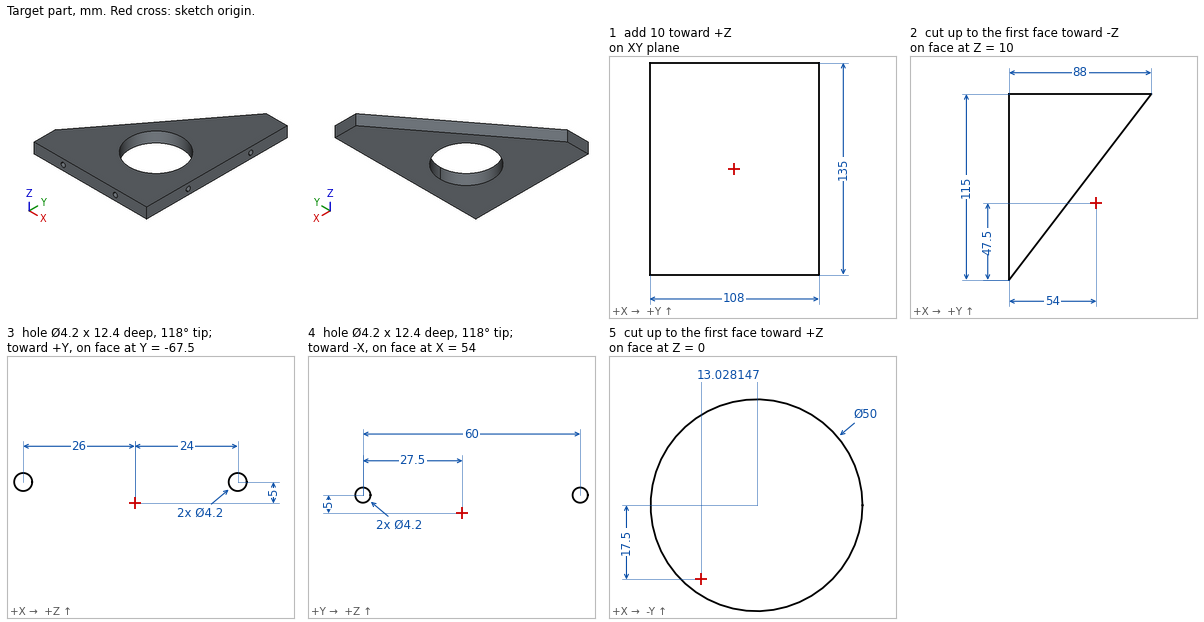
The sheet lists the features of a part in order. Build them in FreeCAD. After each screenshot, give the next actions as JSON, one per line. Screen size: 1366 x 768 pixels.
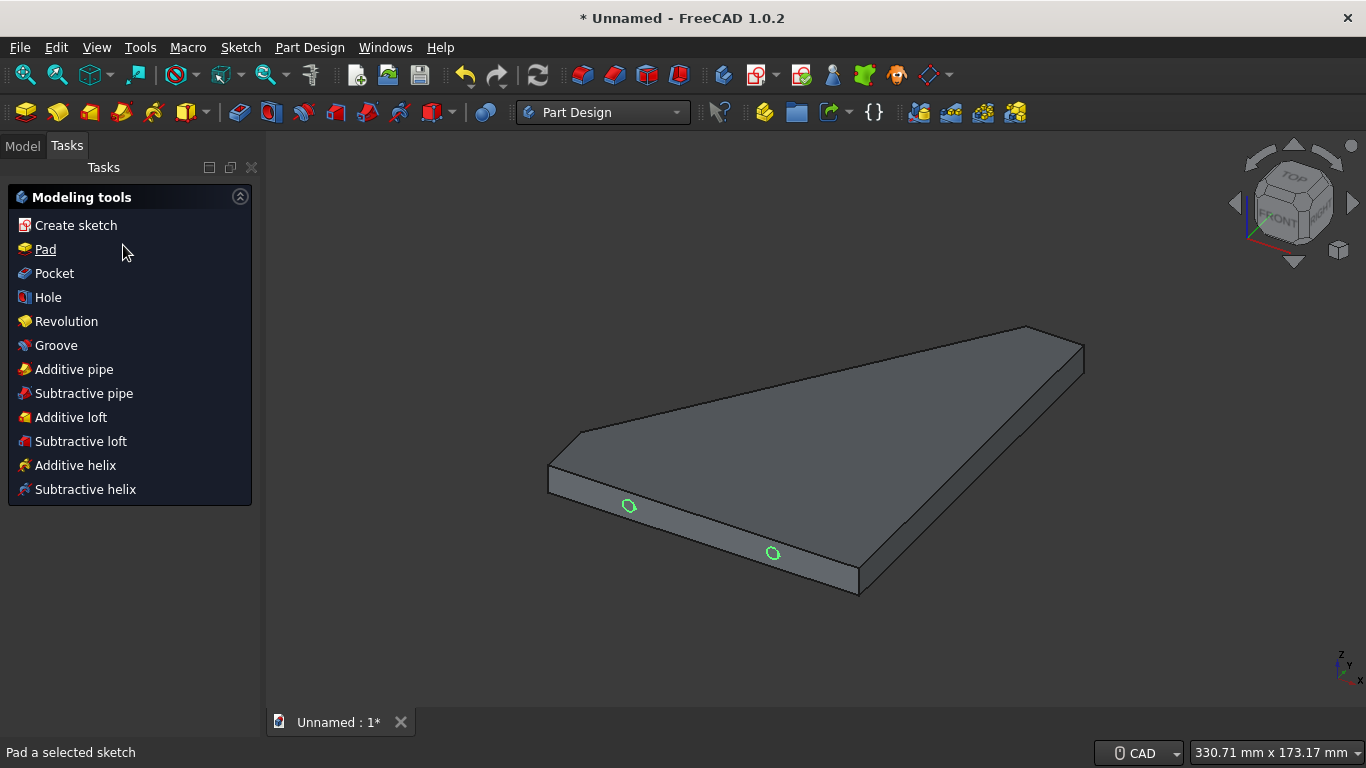
{"action": "left_click", "coordinate": [272, 112]}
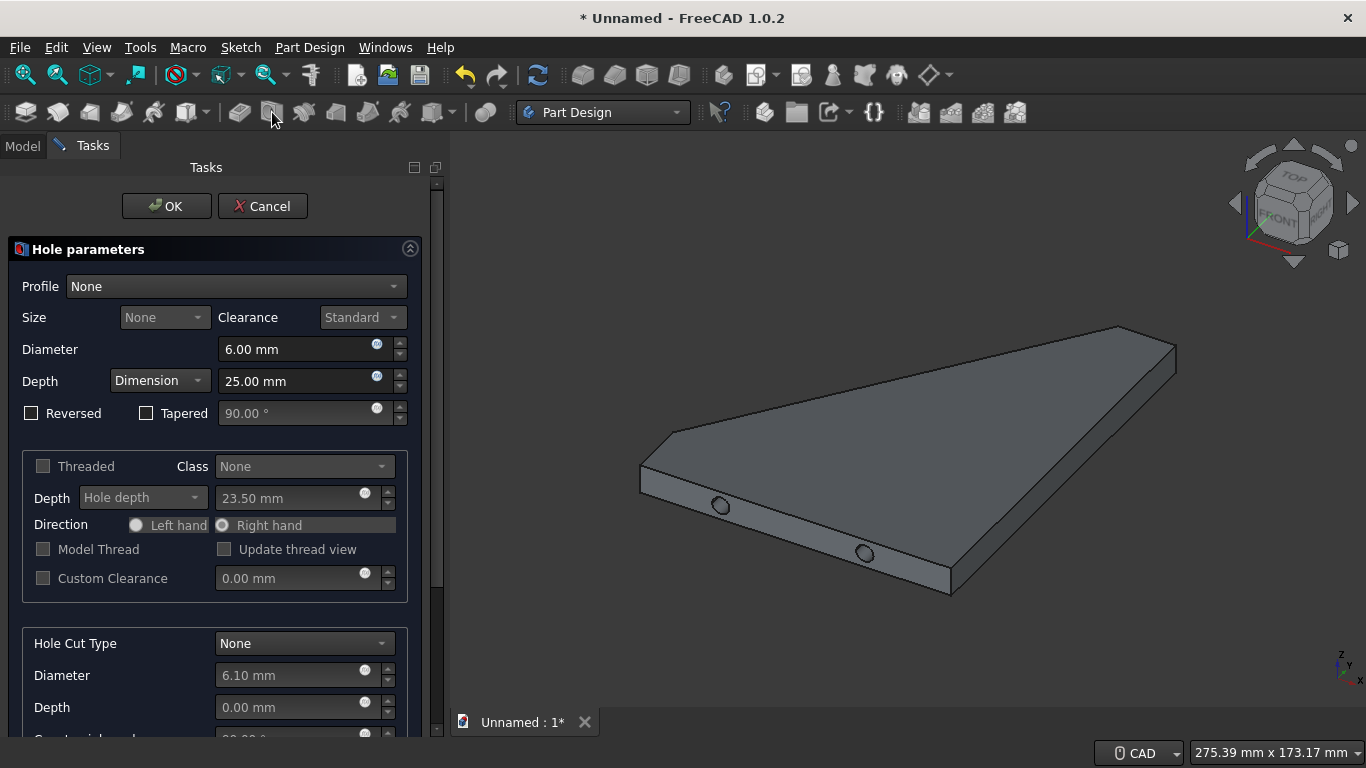
{"action": "triple_click", "coordinate": [305, 349]}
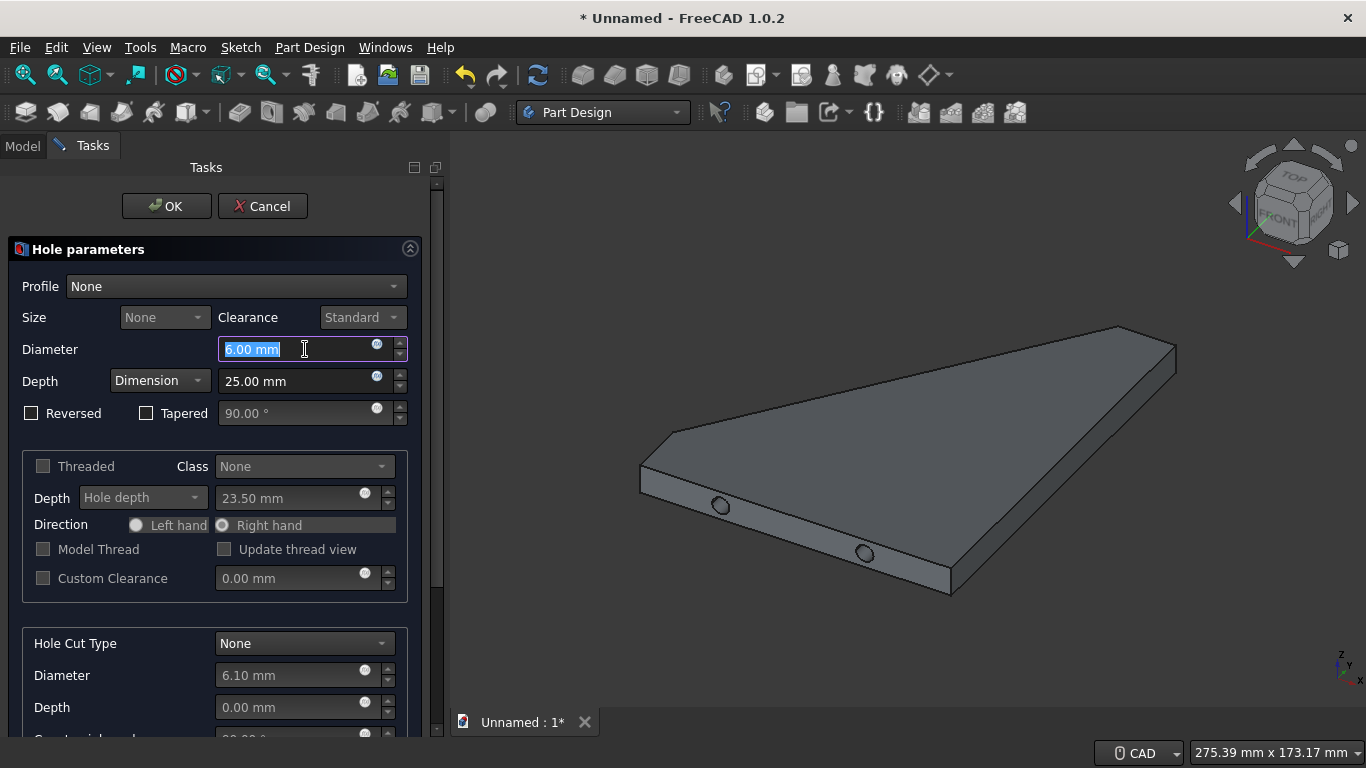
{"action": "type", "text": "4.2"}
{"action": "key", "text": "Tab"}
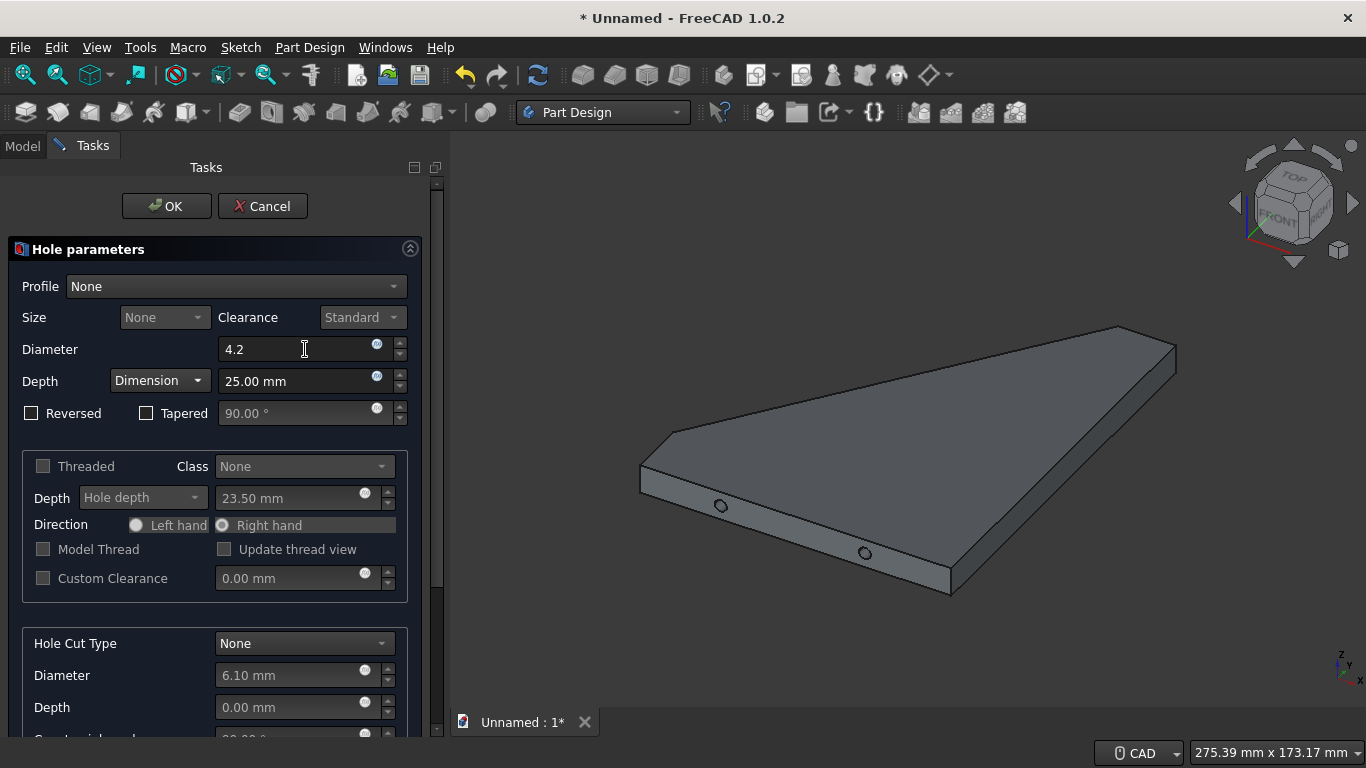
{"action": "triple_click", "coordinate": [305, 381]}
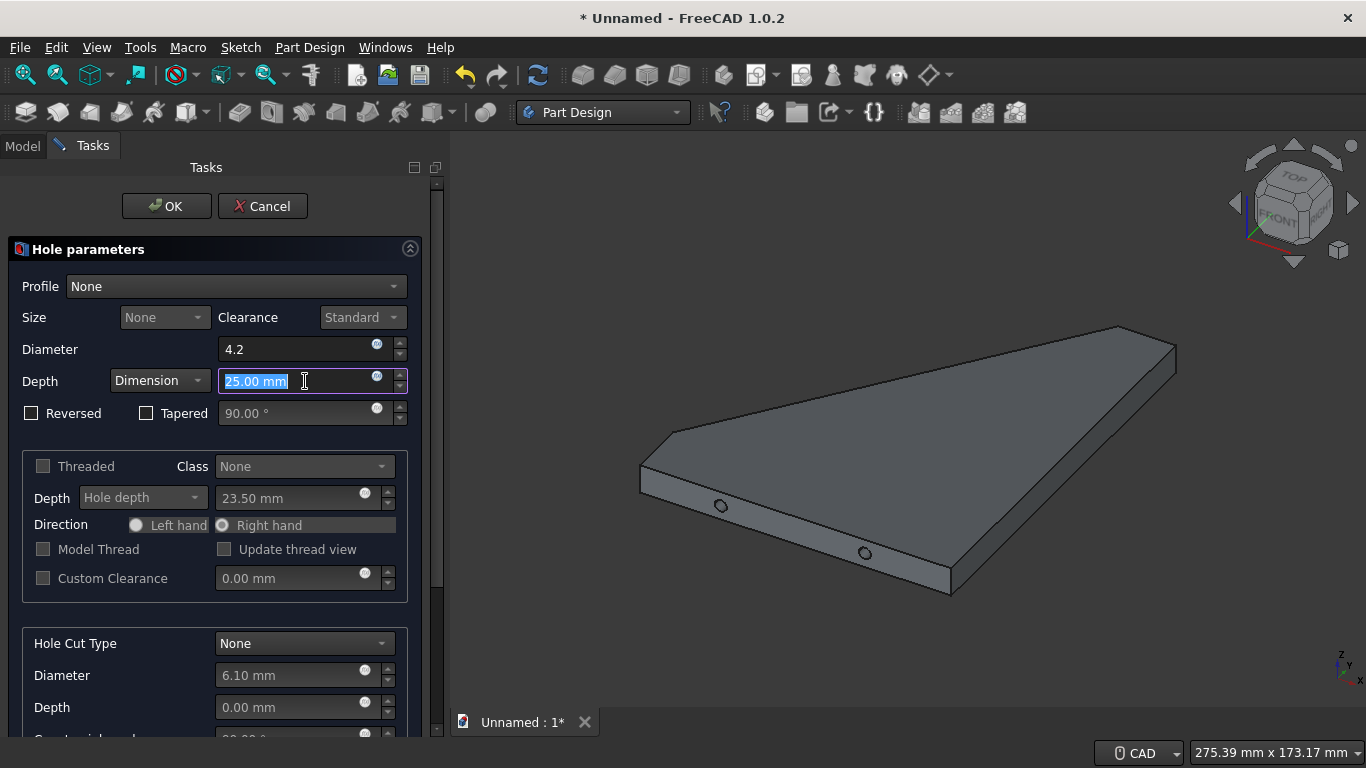
{"action": "type", "text": "12.4"}
{"action": "key", "text": "Tab"}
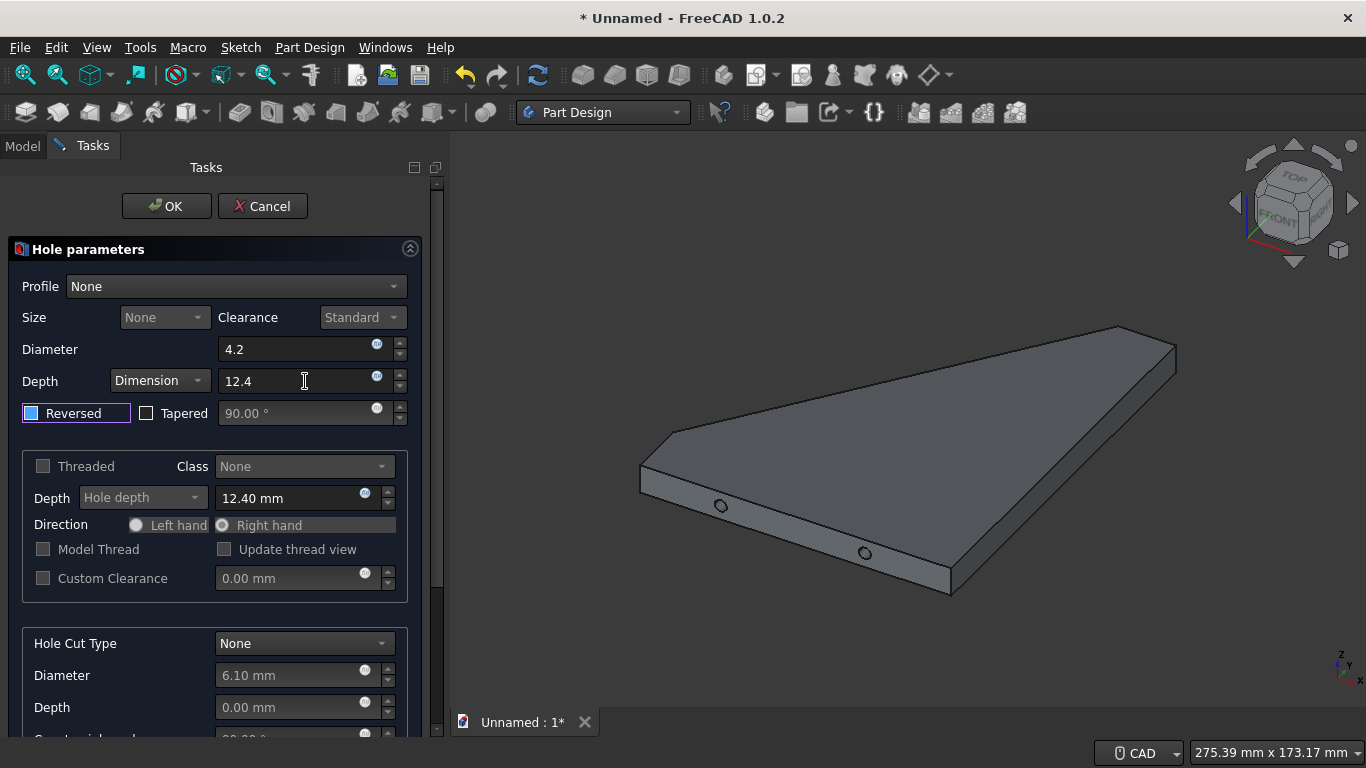
{"action": "left_click", "coordinate": [167, 206]}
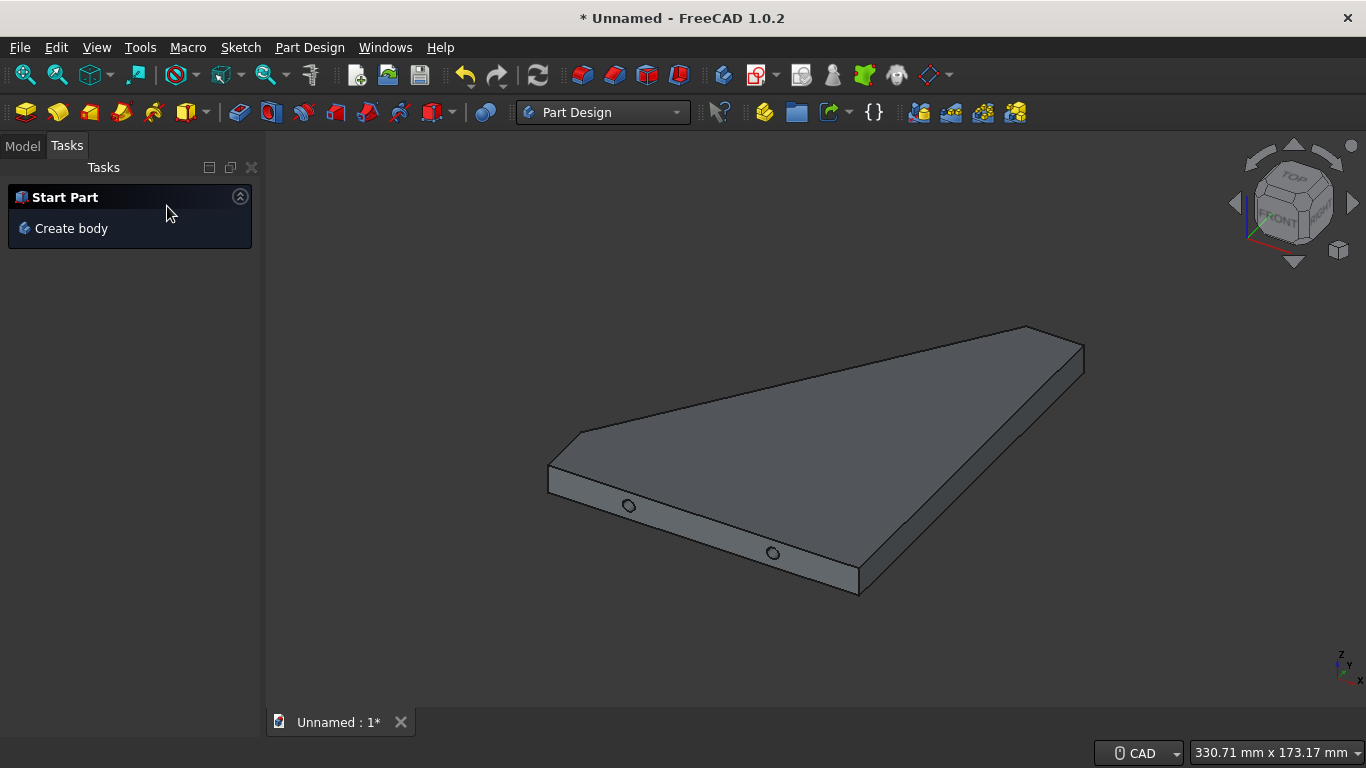
{"action": "left_click", "coordinate": [1068, 374]}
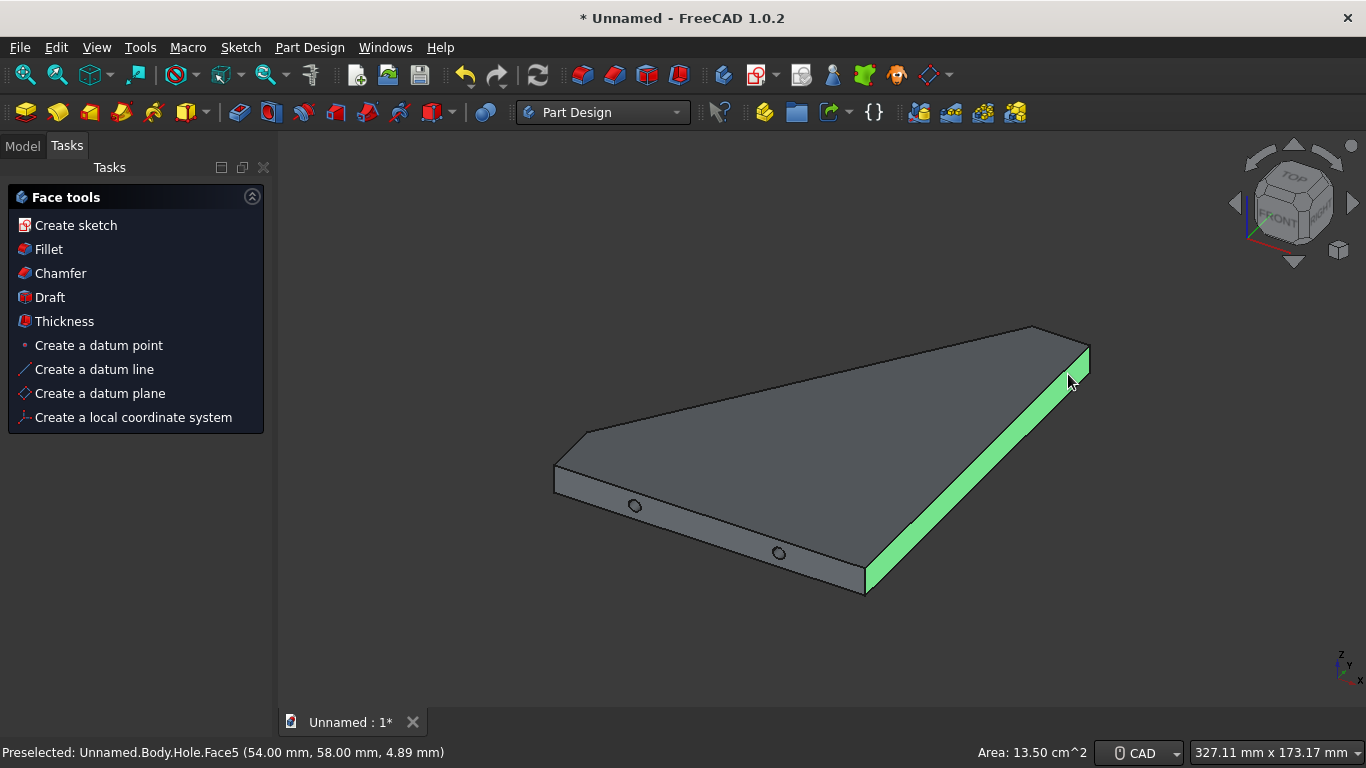
{"action": "left_click", "coordinate": [756, 76]}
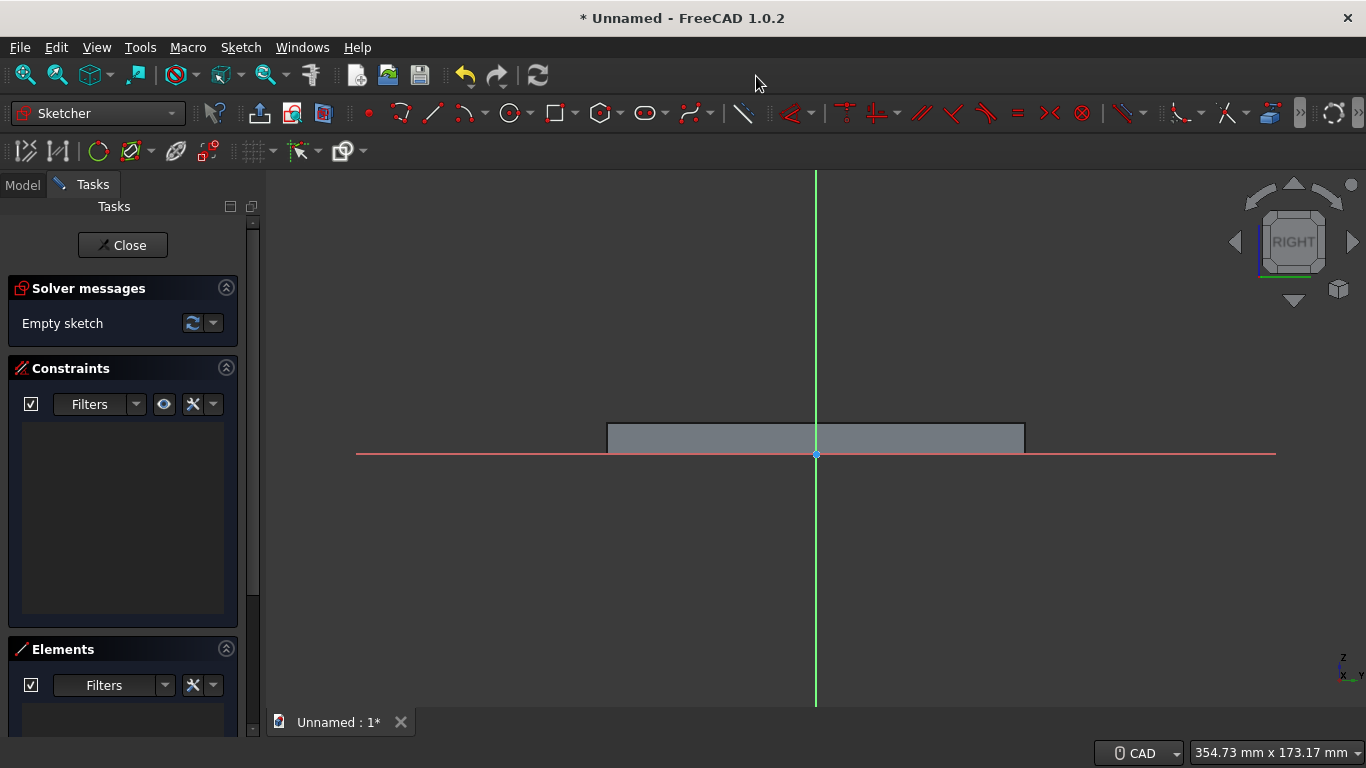
{"action": "scroll", "coordinate": [857, 445], "scroll_direction": "up", "scroll_amount": 6}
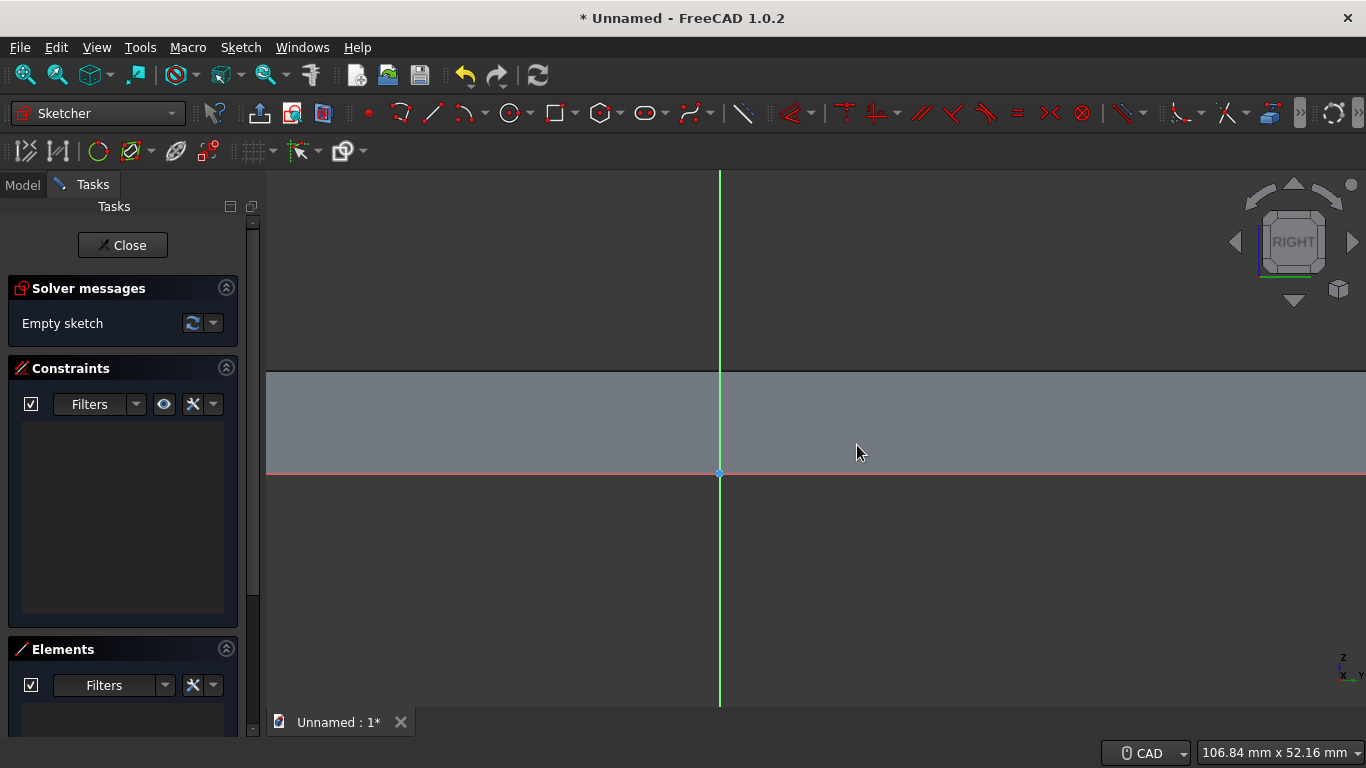
{"action": "key", "text": "g c"}